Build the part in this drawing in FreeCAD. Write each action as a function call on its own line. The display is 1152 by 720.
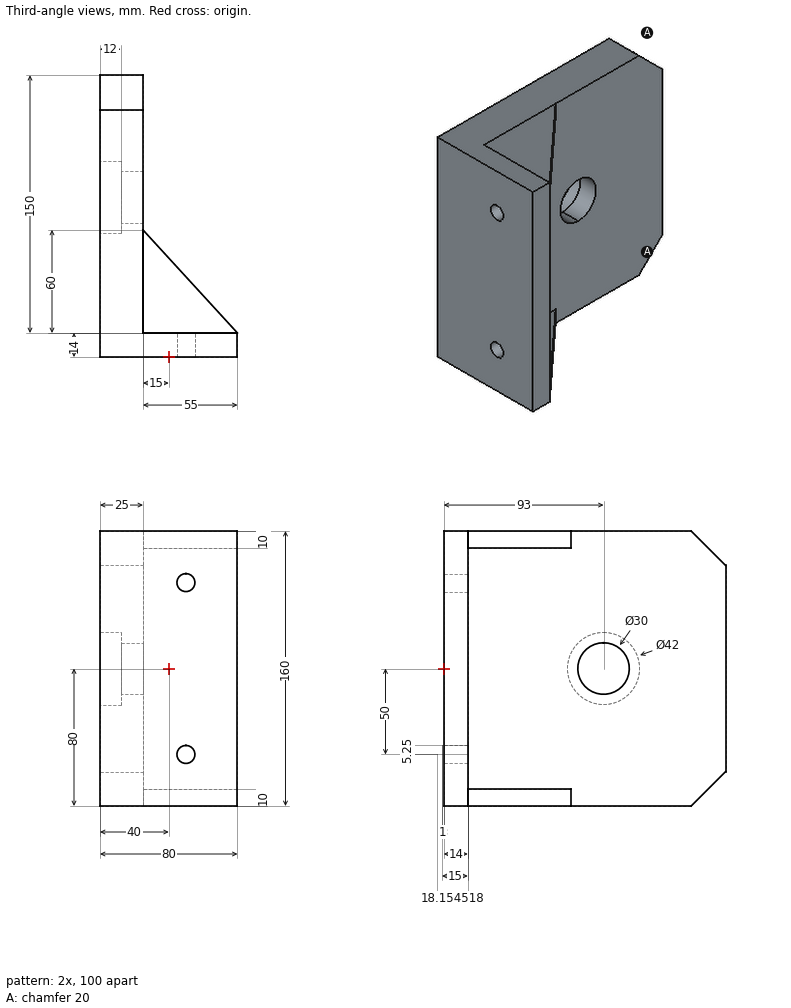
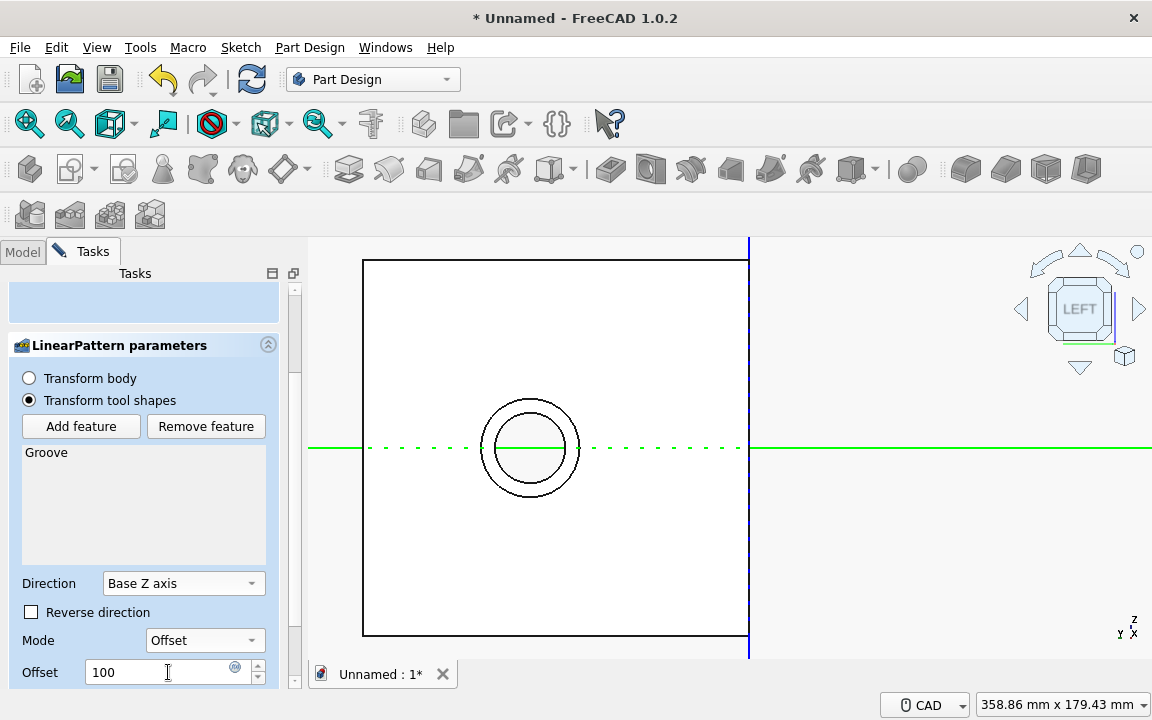
scroll(295, 486, down, 2)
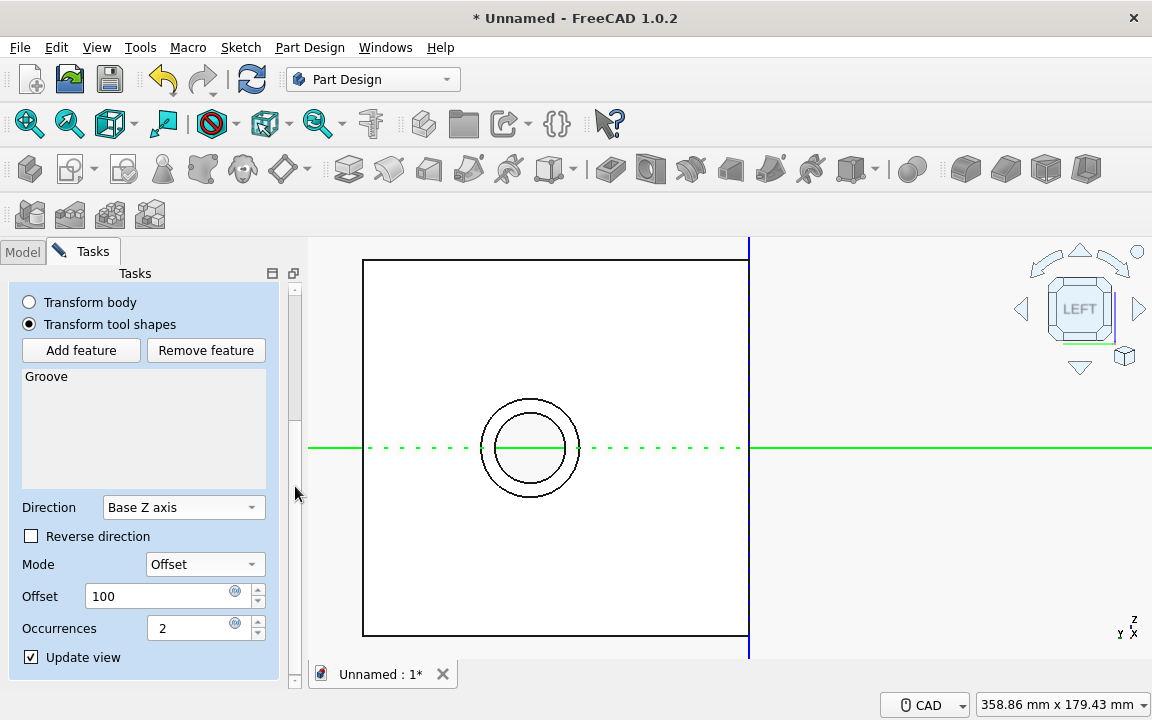
triple_click(198, 628)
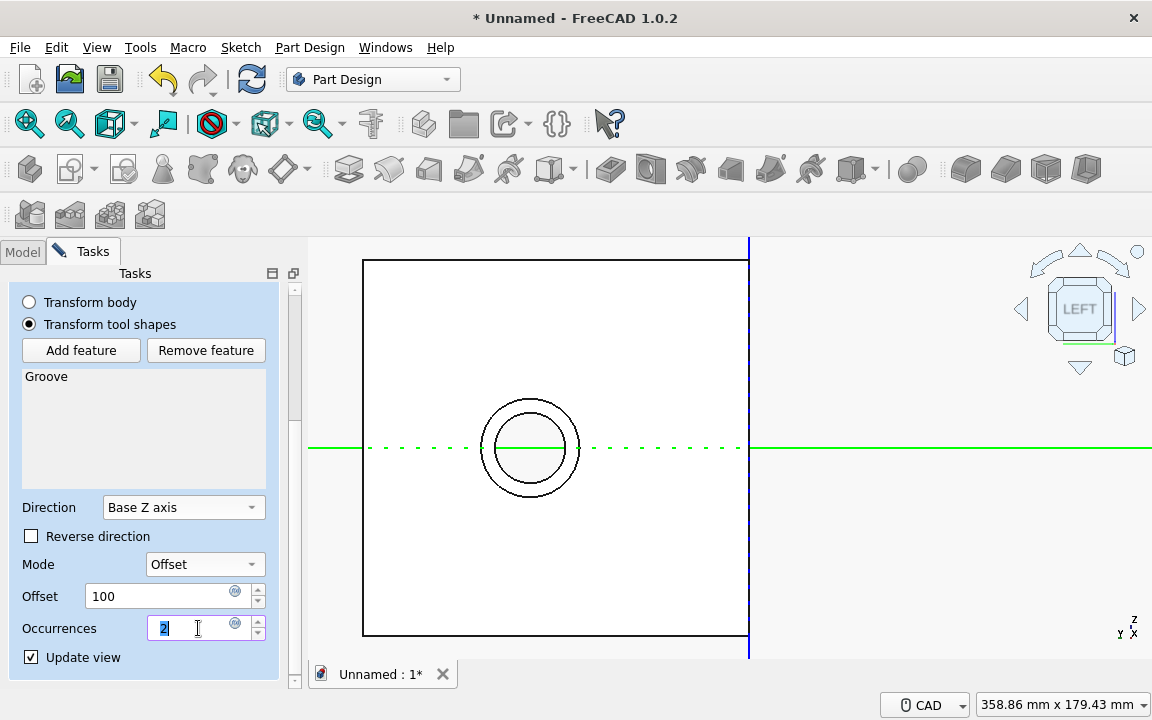
text(2)
key(Tab)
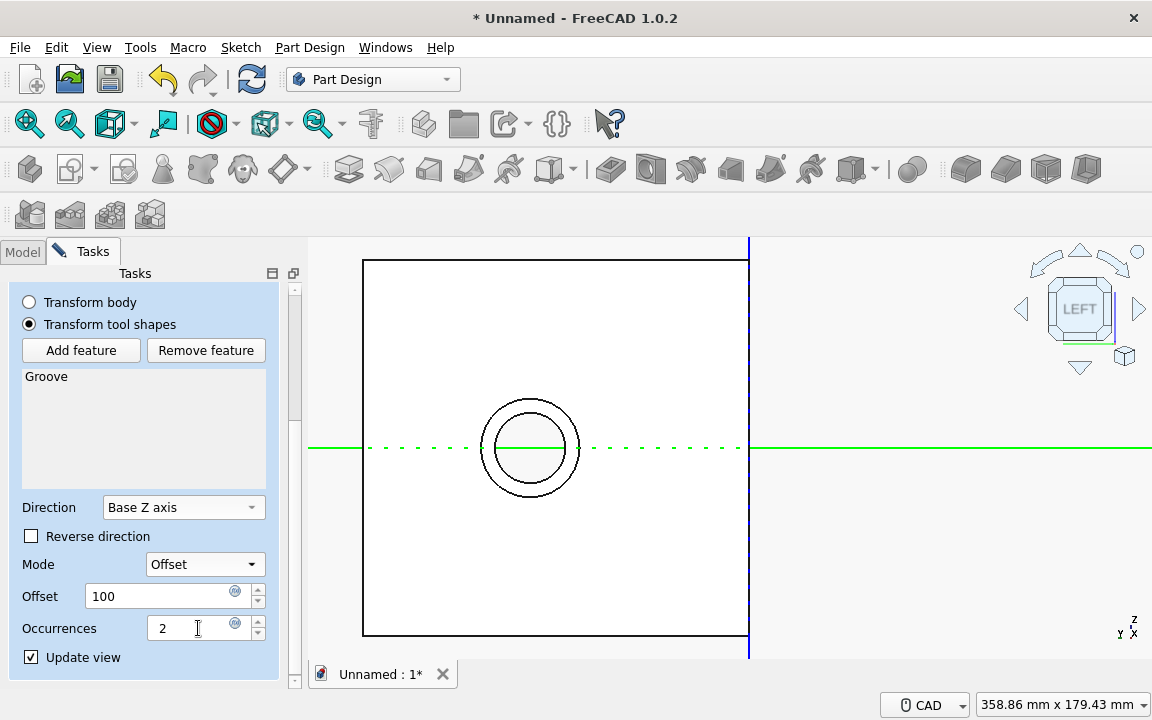
scroll(295, 486, up, 5)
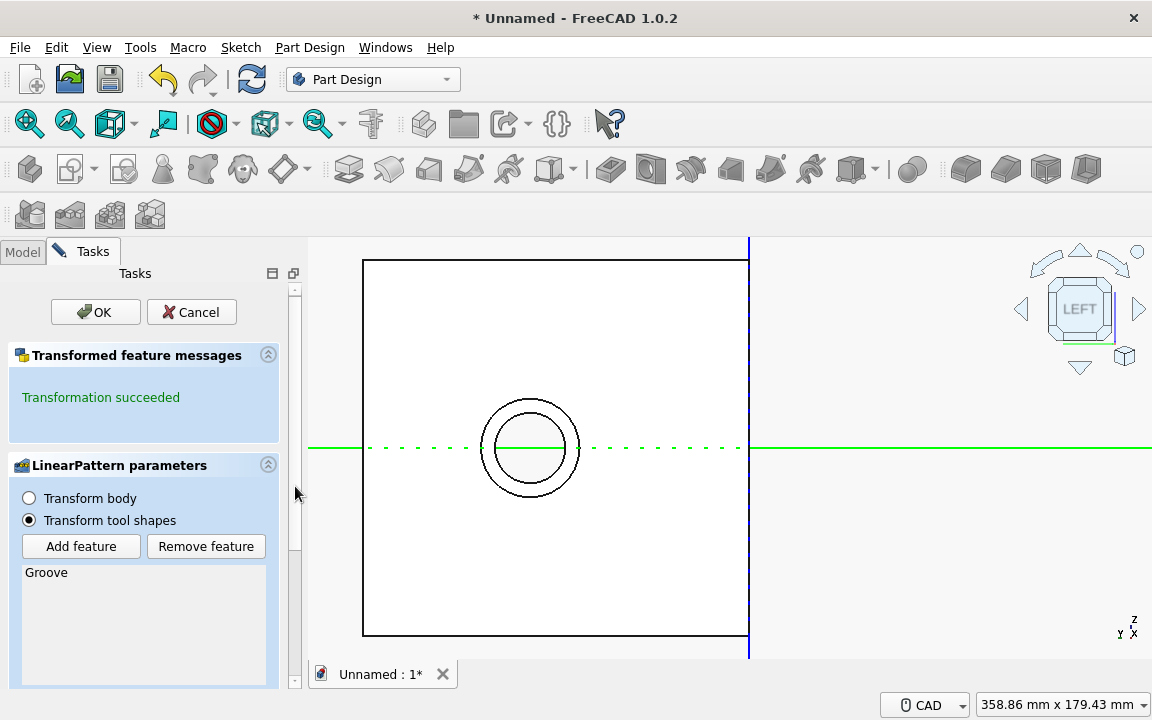
click(96, 312)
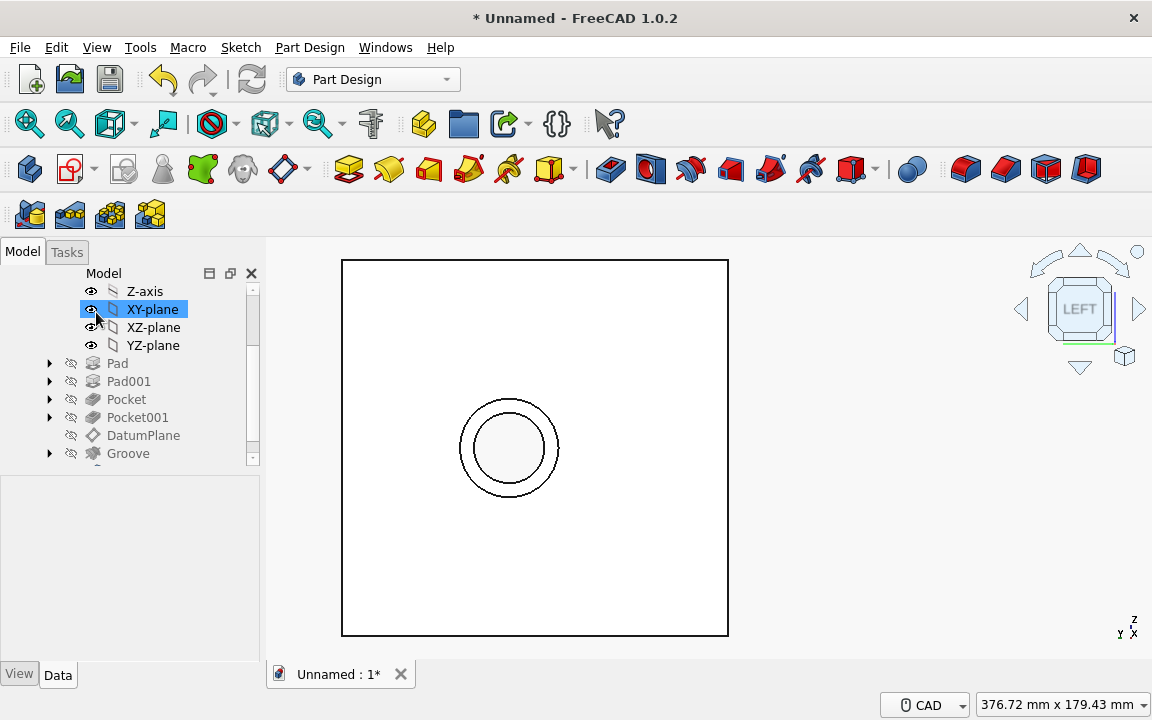
key(0)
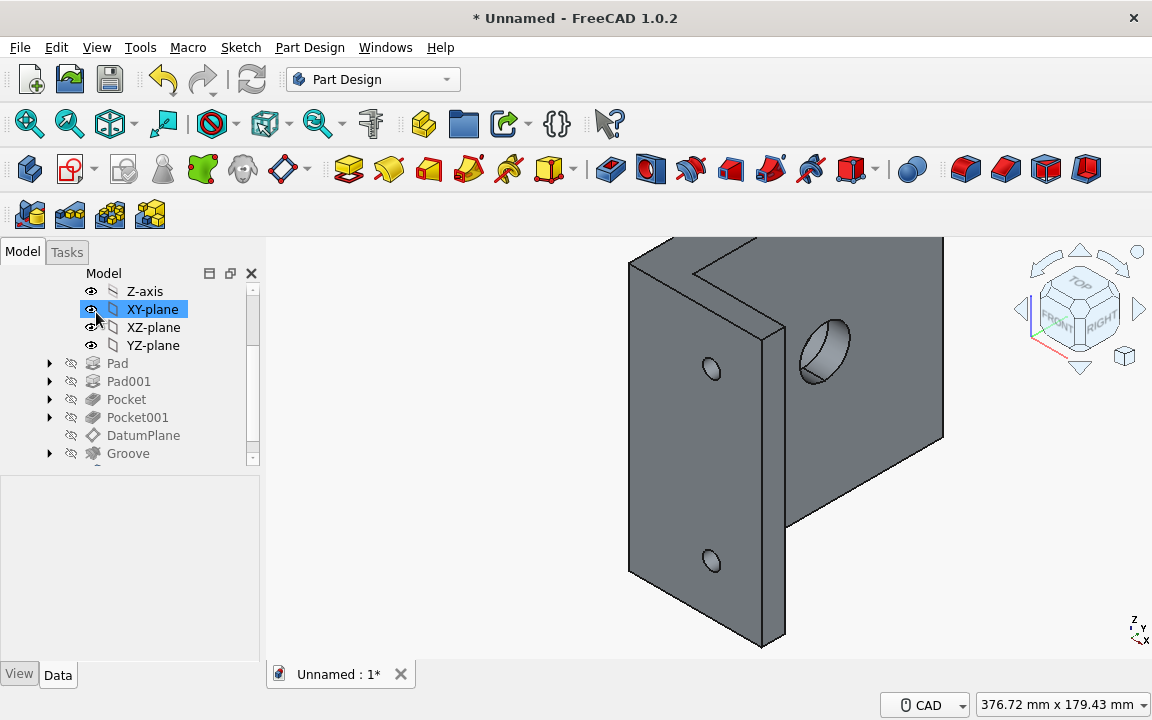
click(30, 124)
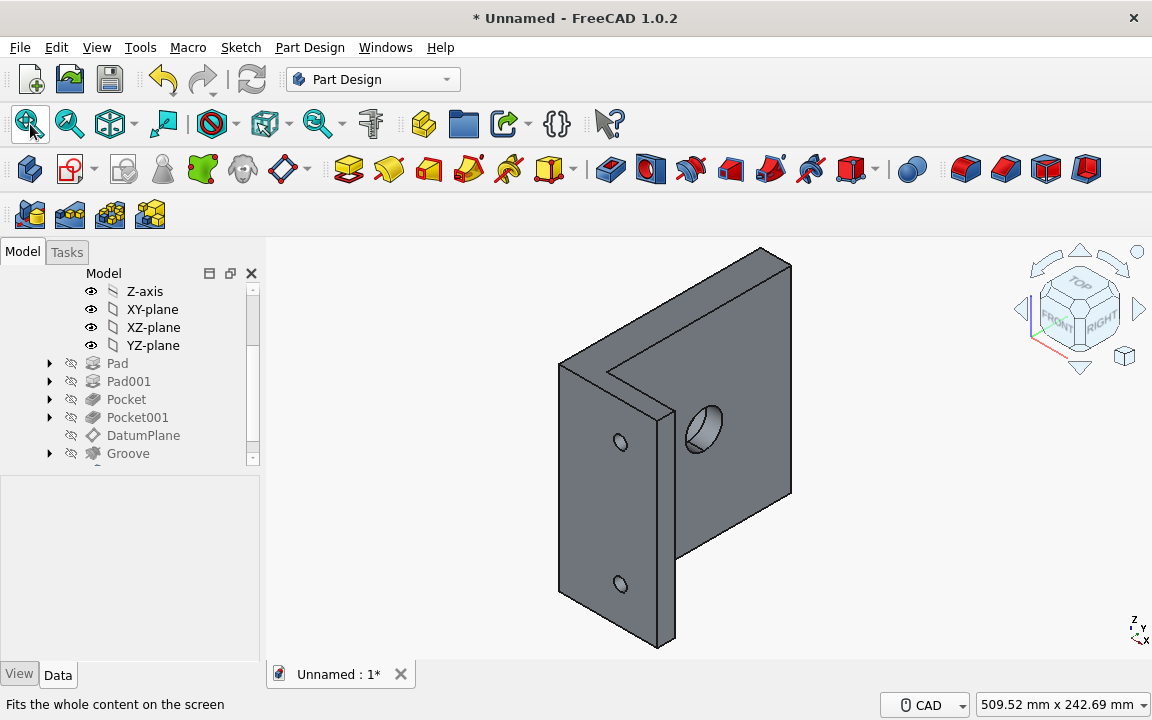
key(2)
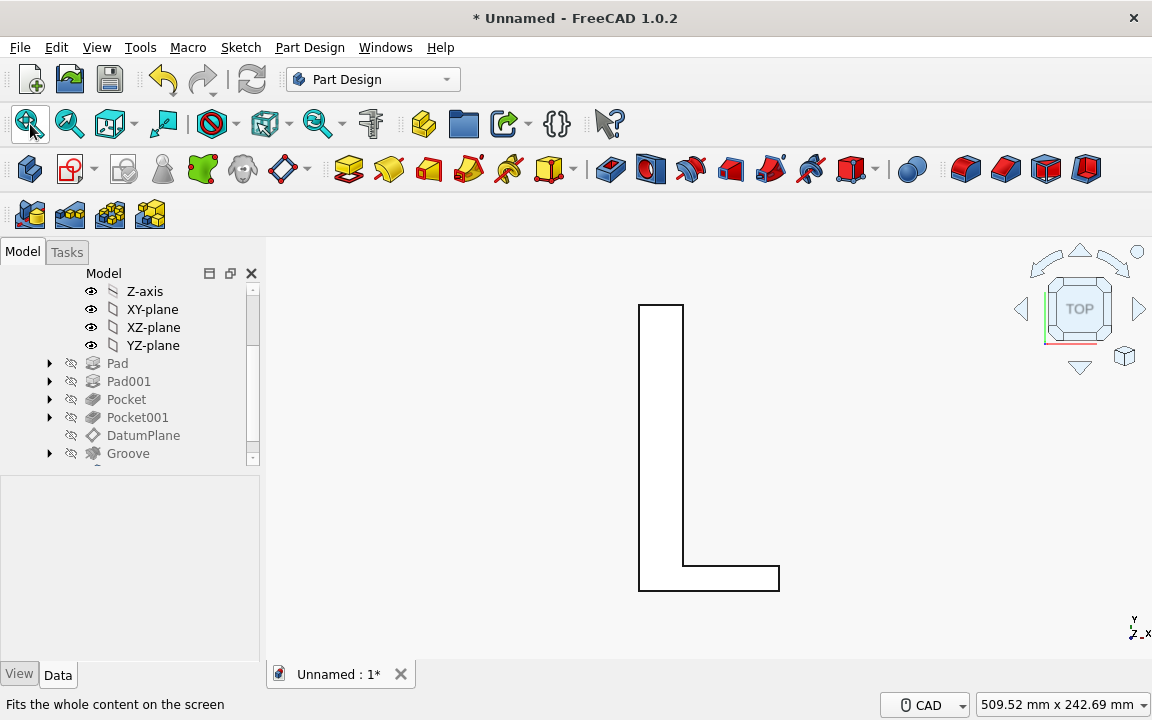
click(661, 304)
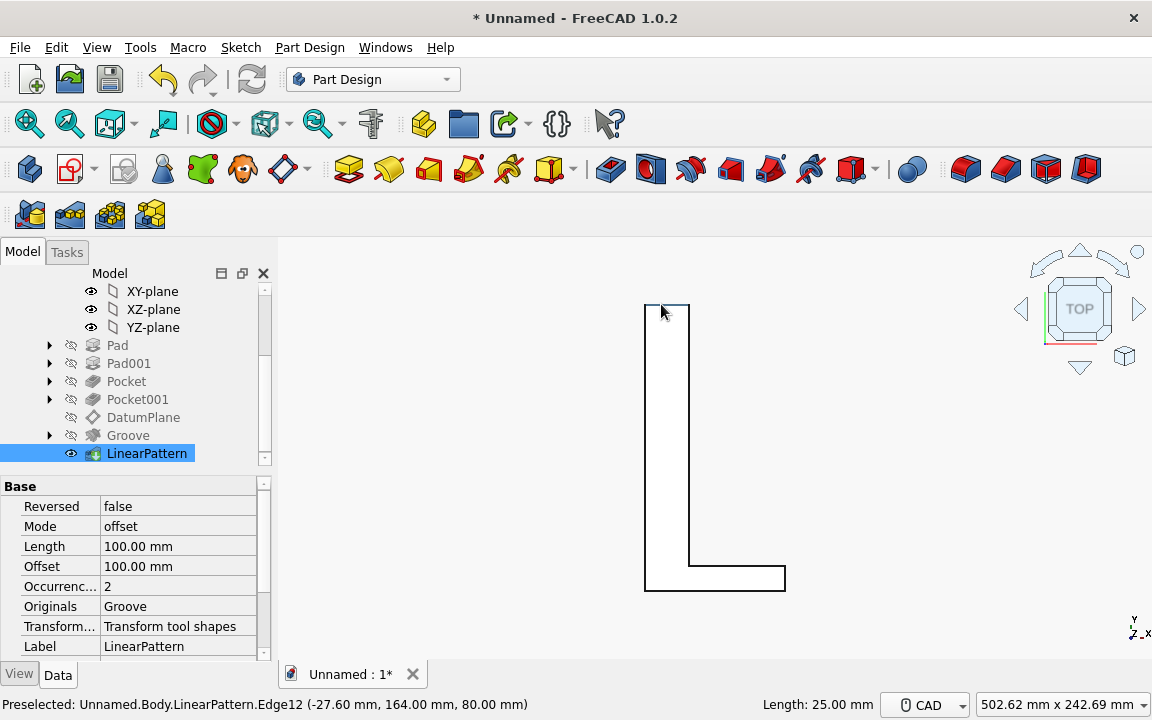
key(1)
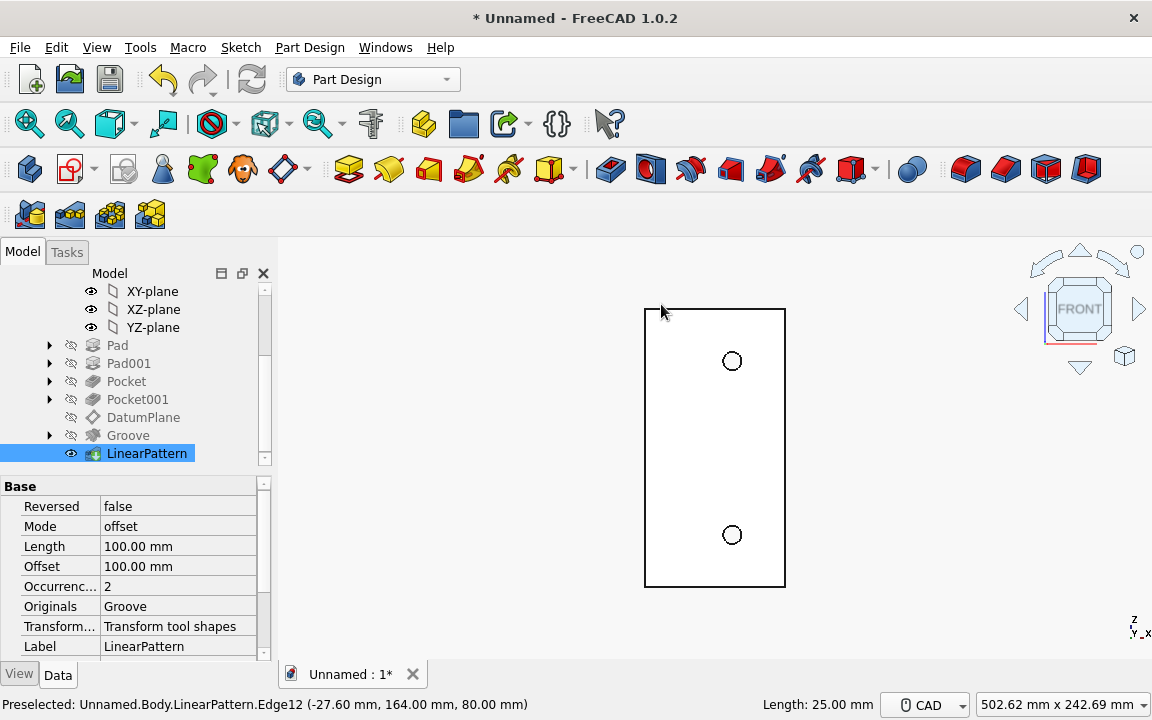
key(3)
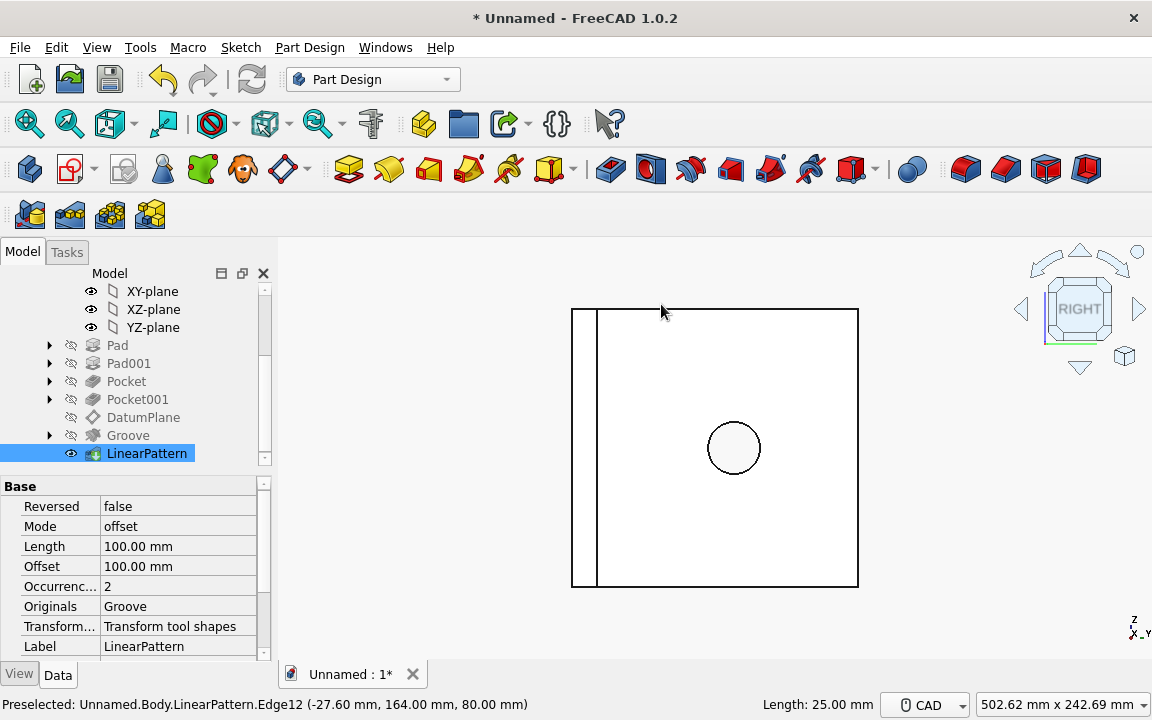
key(5)